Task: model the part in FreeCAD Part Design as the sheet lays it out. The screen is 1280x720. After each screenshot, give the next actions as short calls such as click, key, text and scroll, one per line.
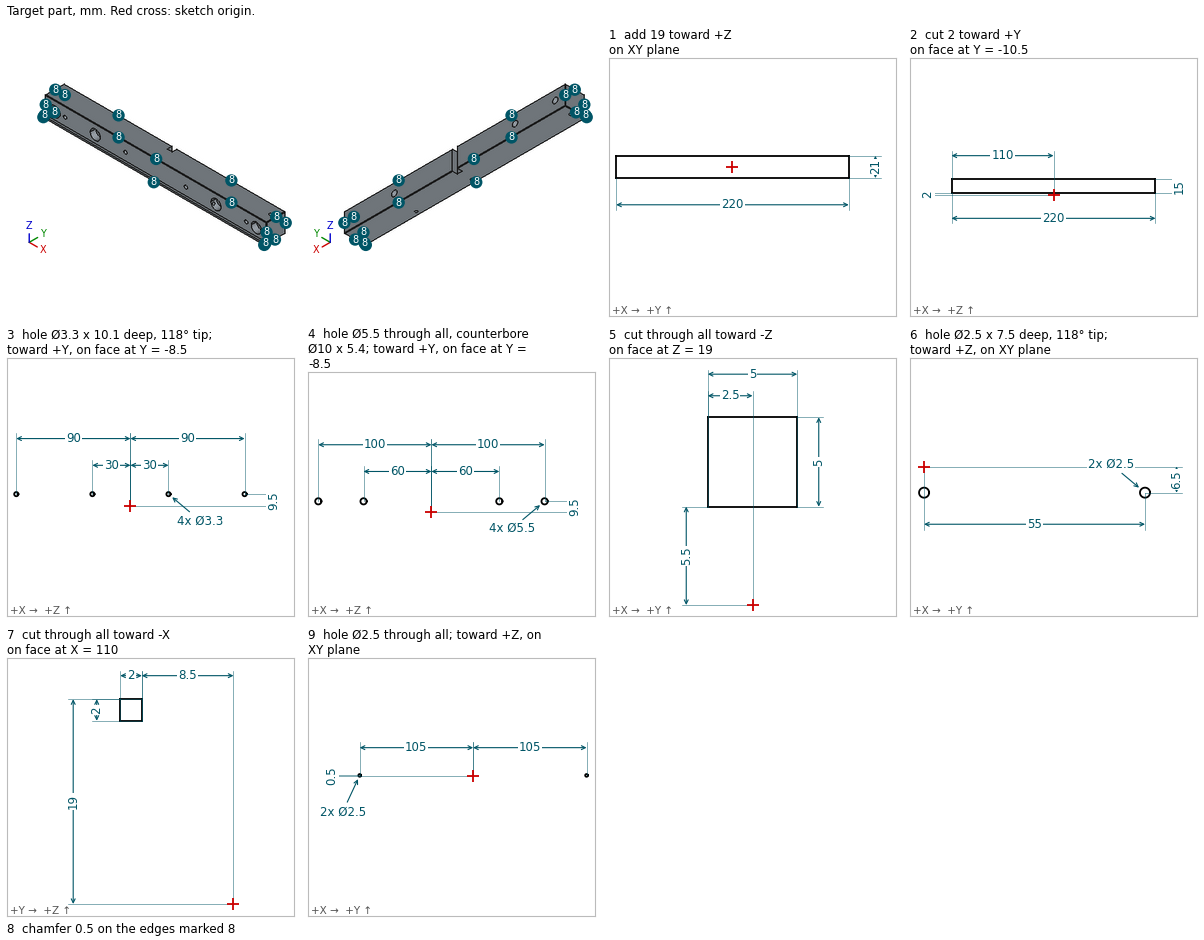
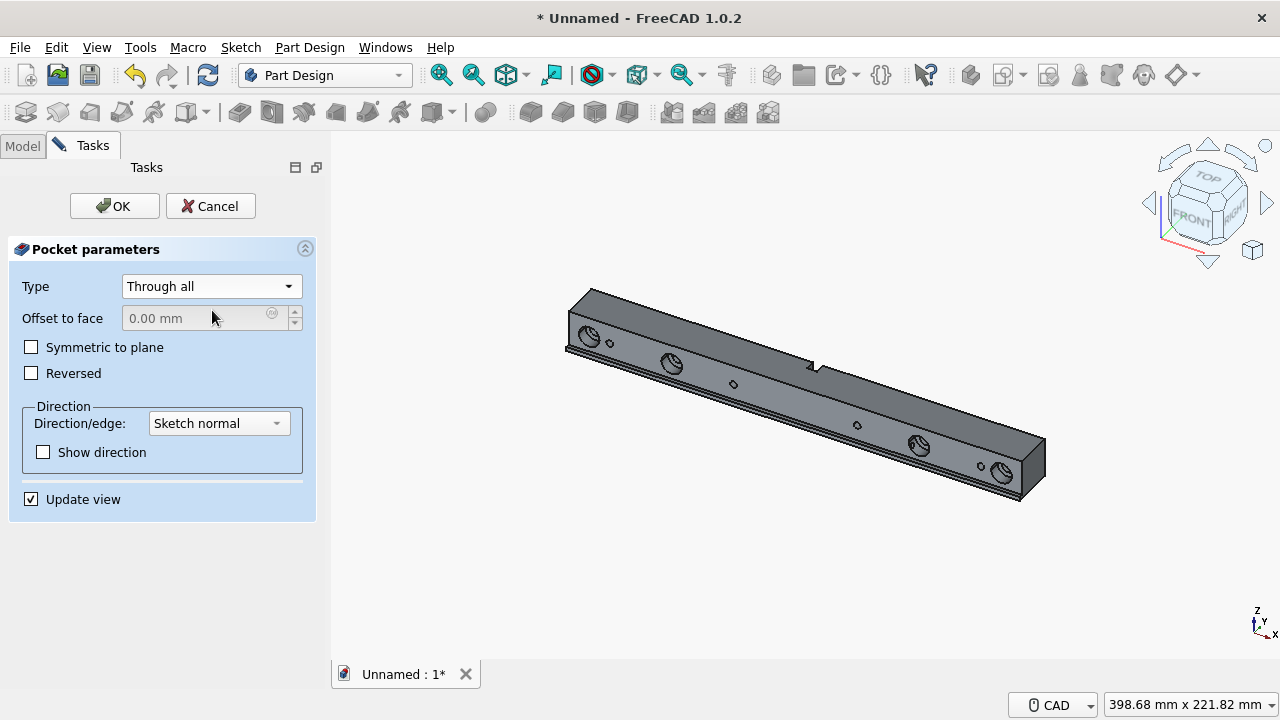
click(115, 206)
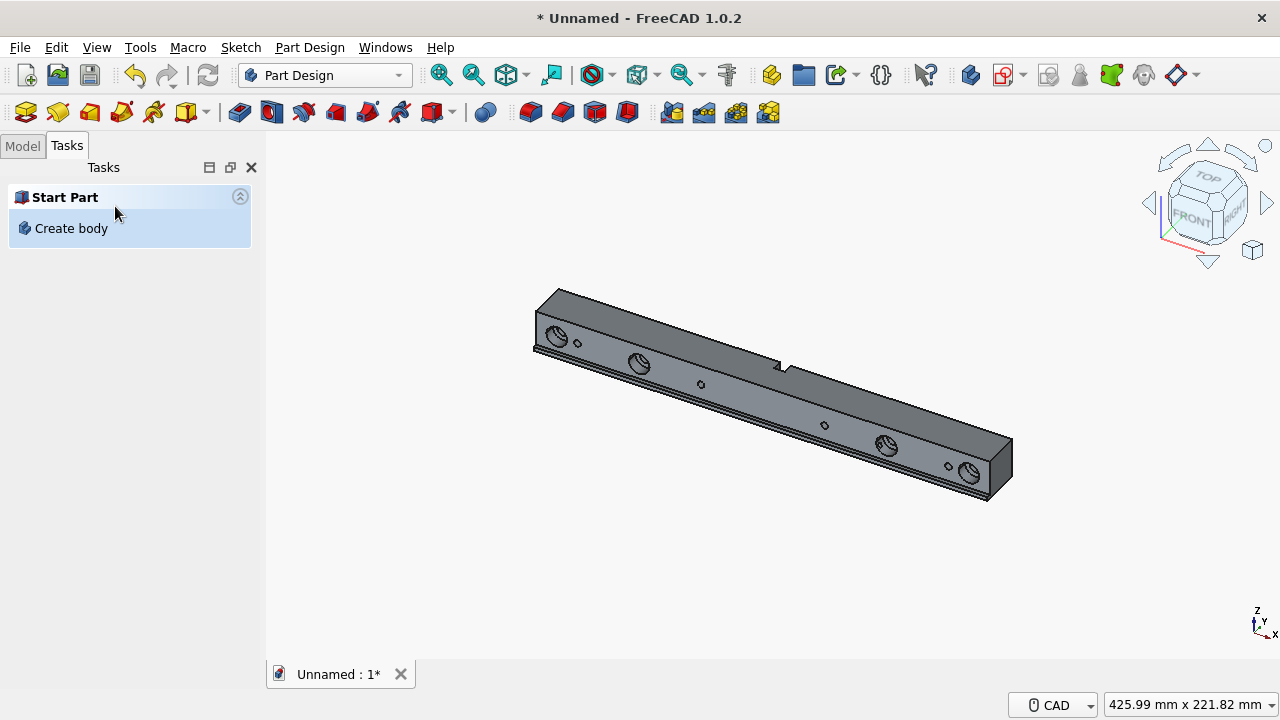
click(1000, 469)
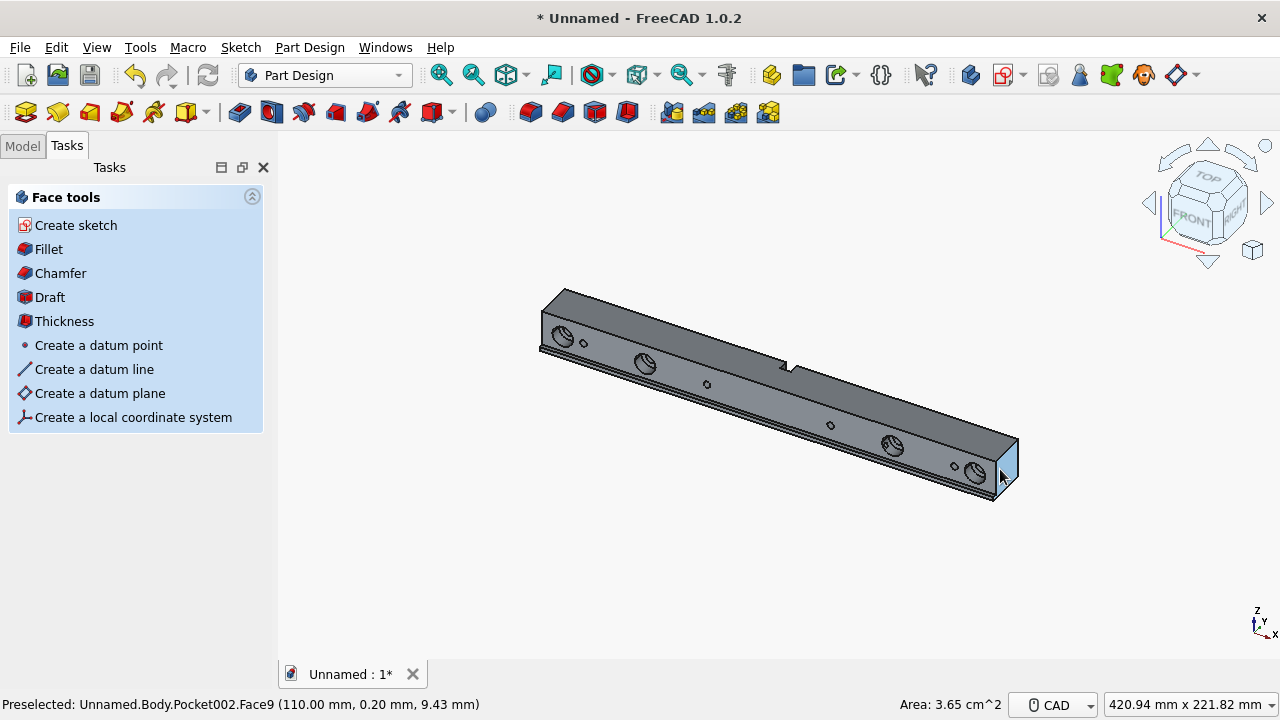
click(769, 386, ctrl)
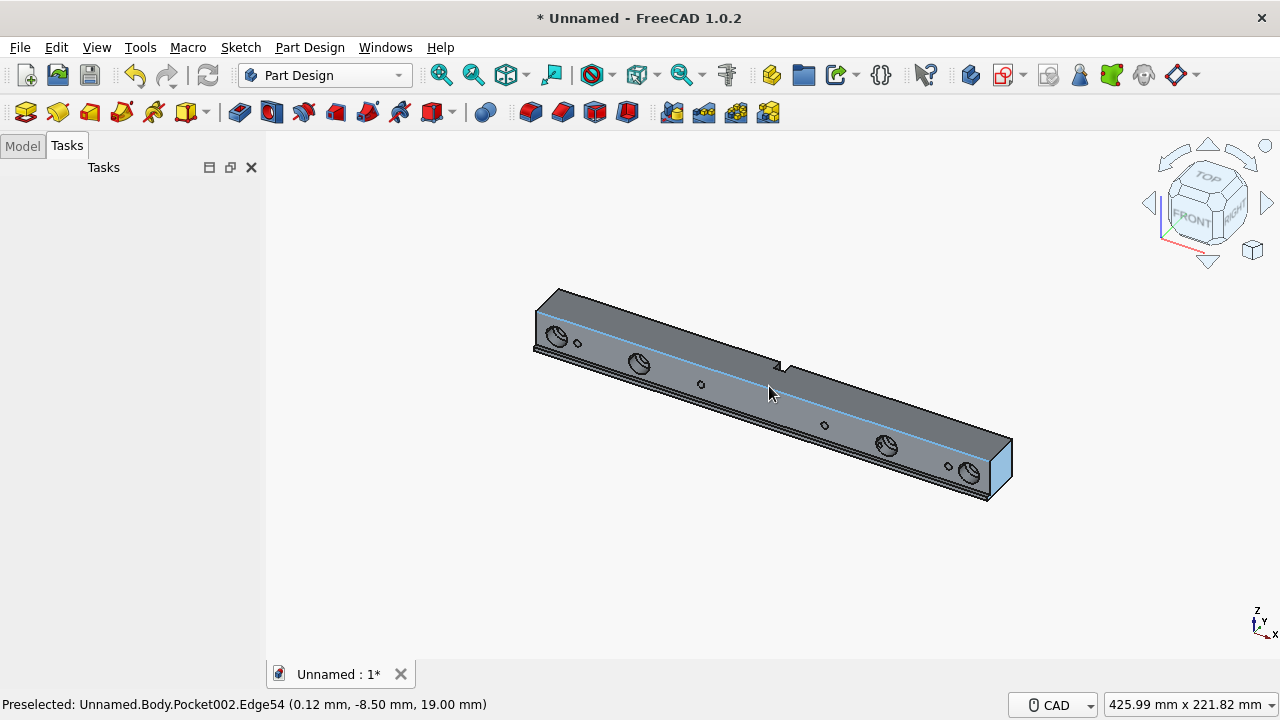
key(0)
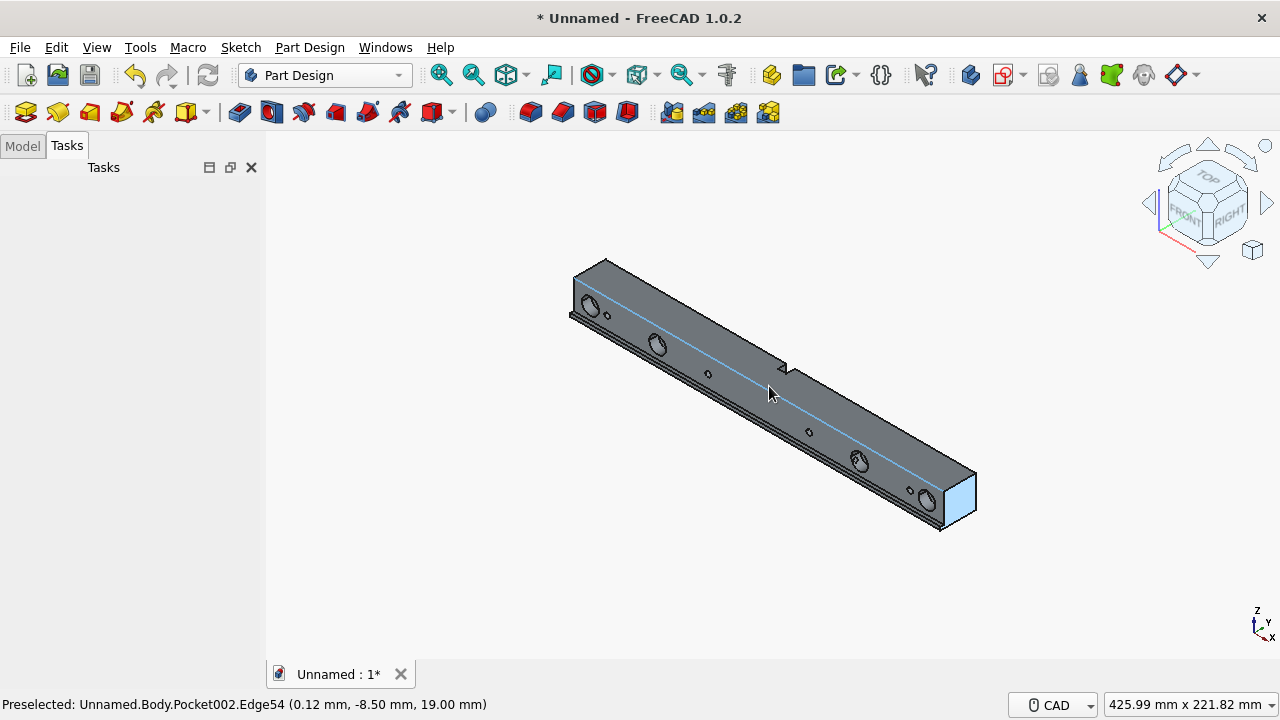
key(2)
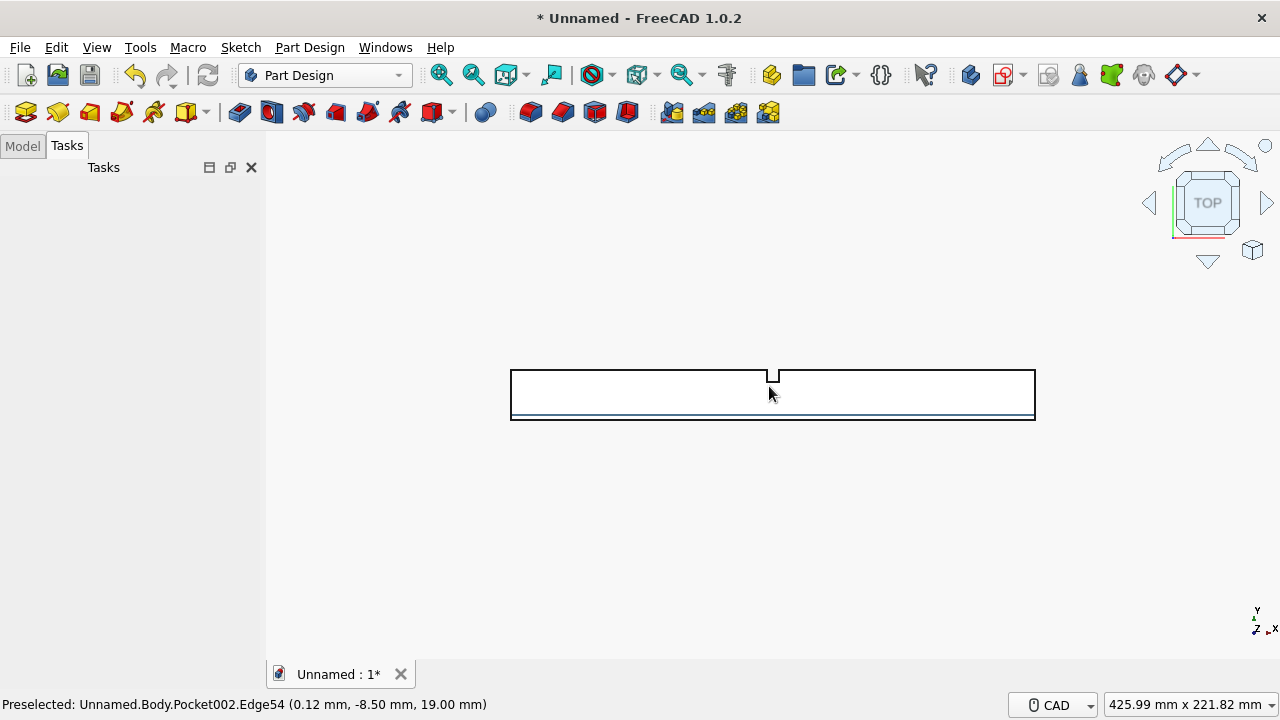
click(907, 369, ctrl)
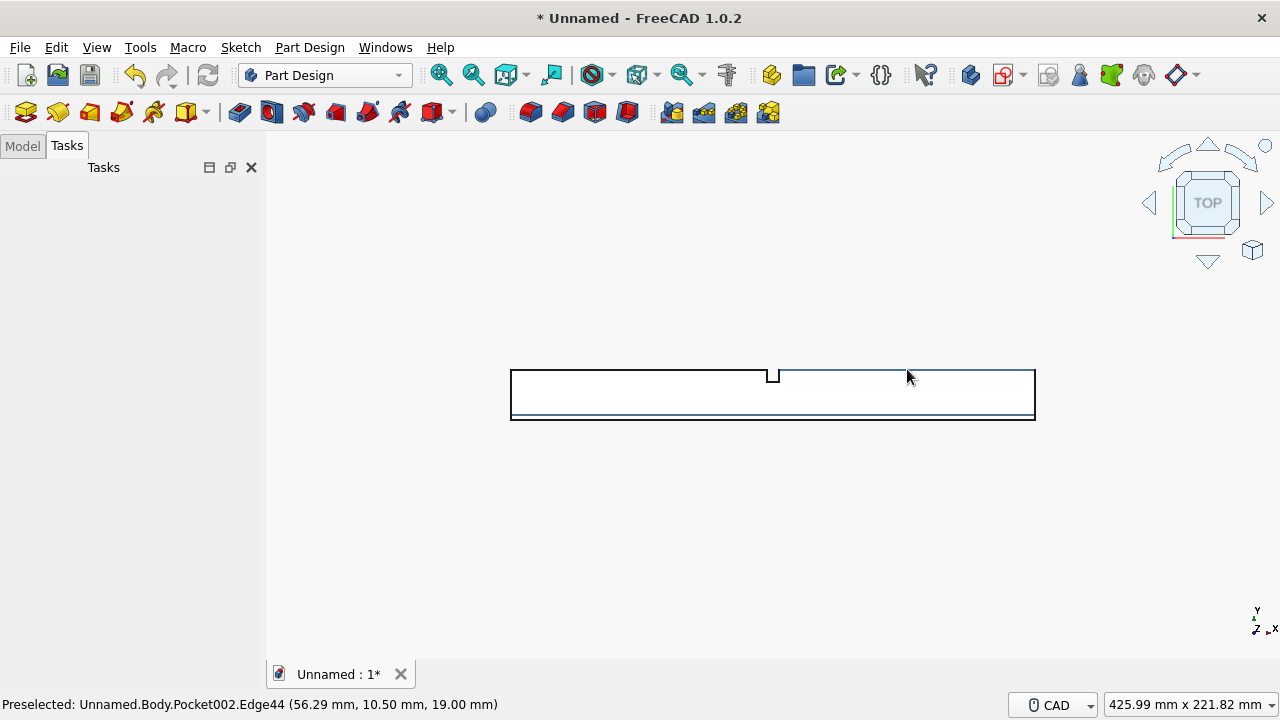
click(639, 369, ctrl)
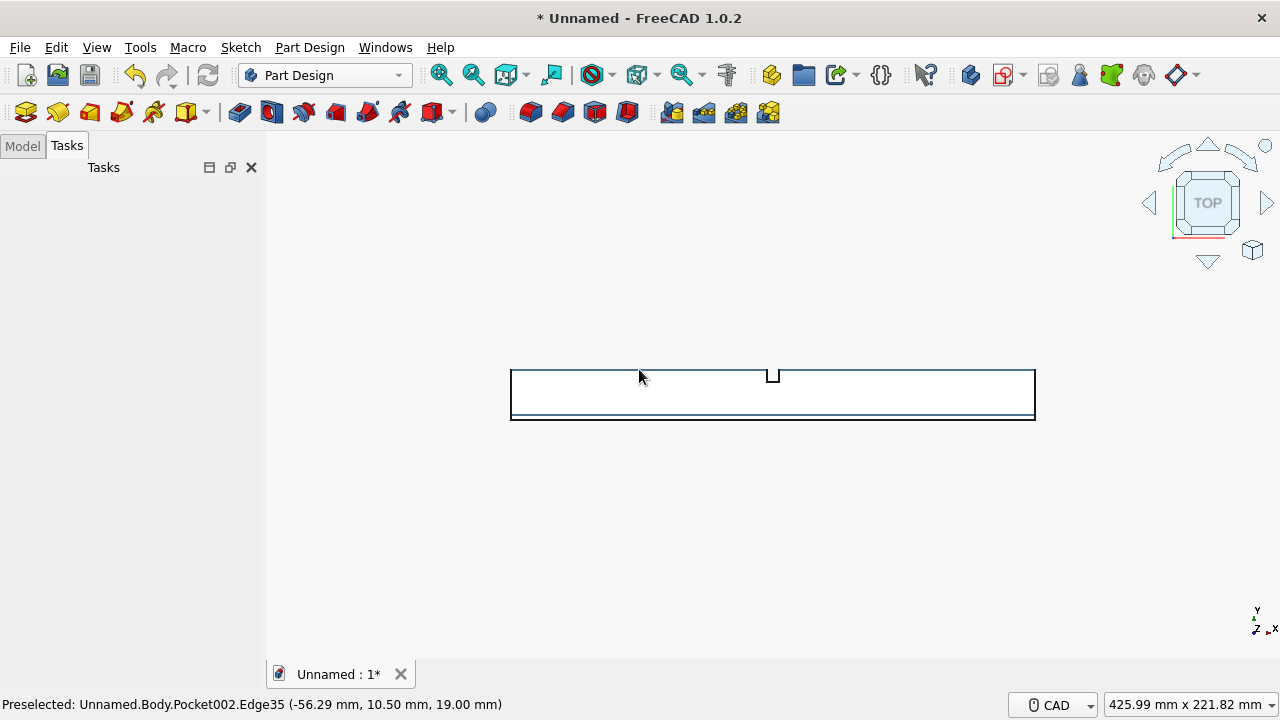
key(1)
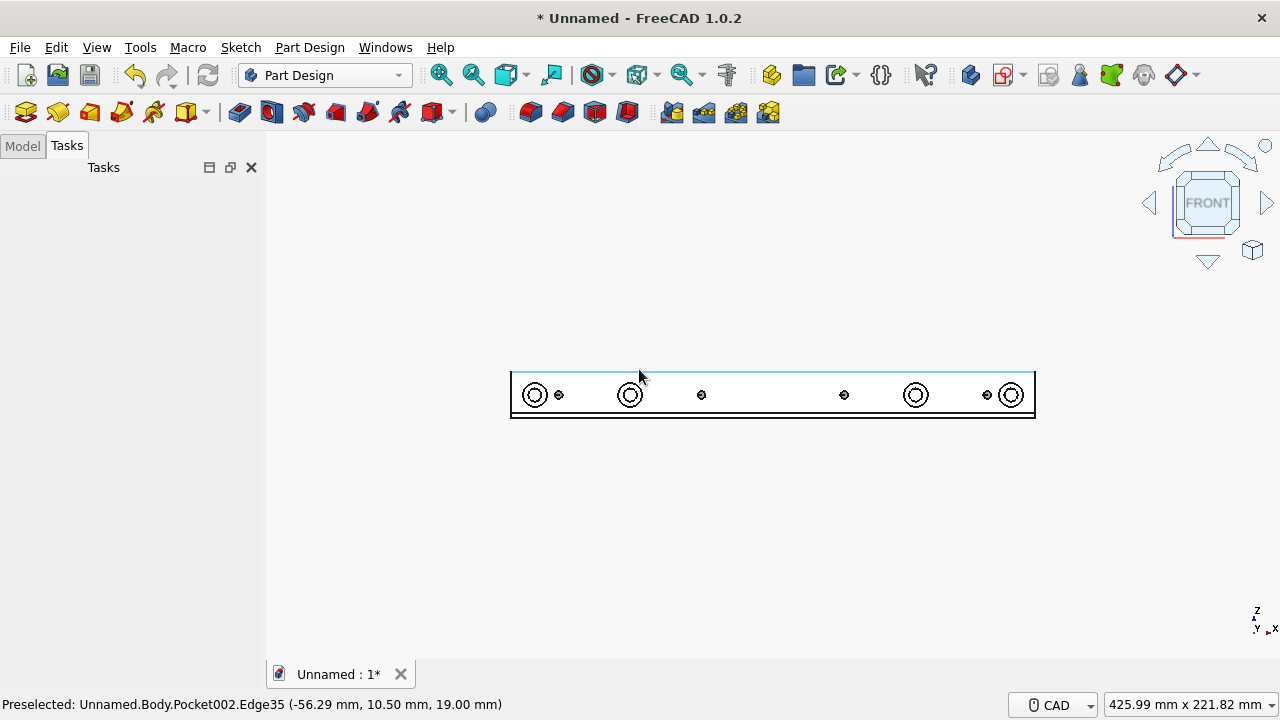
click(773, 417, ctrl)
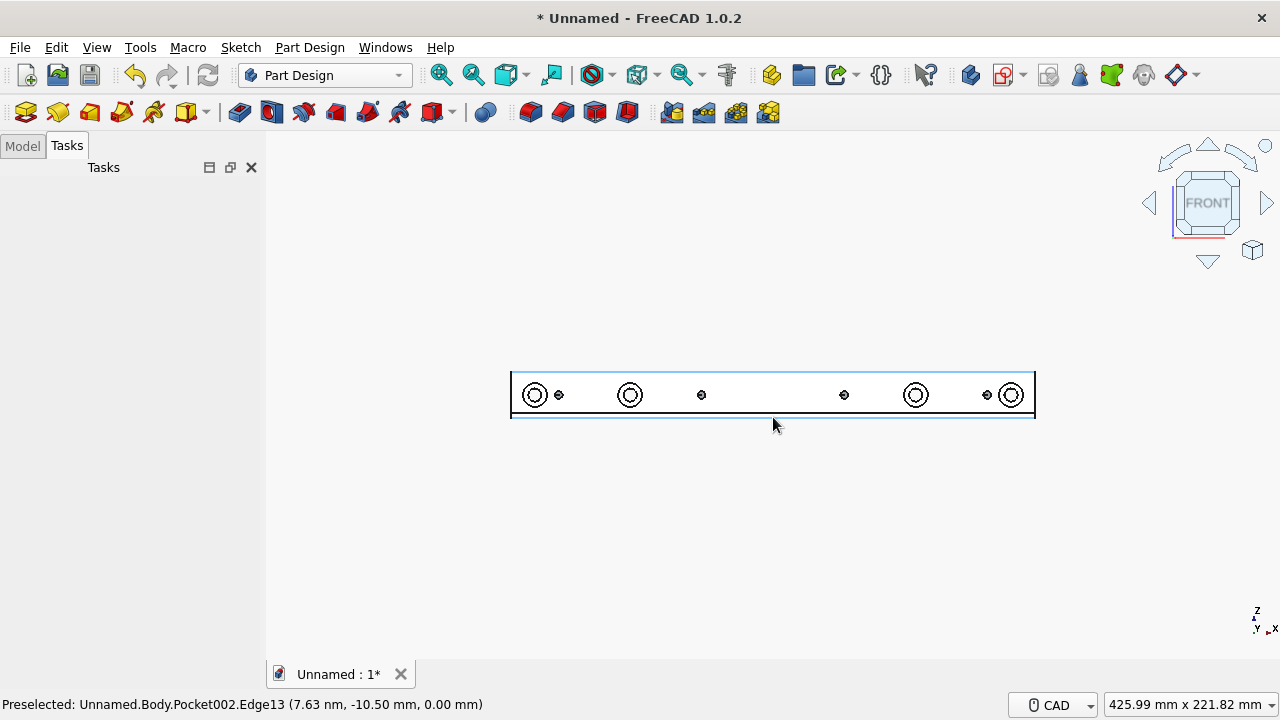
key(3)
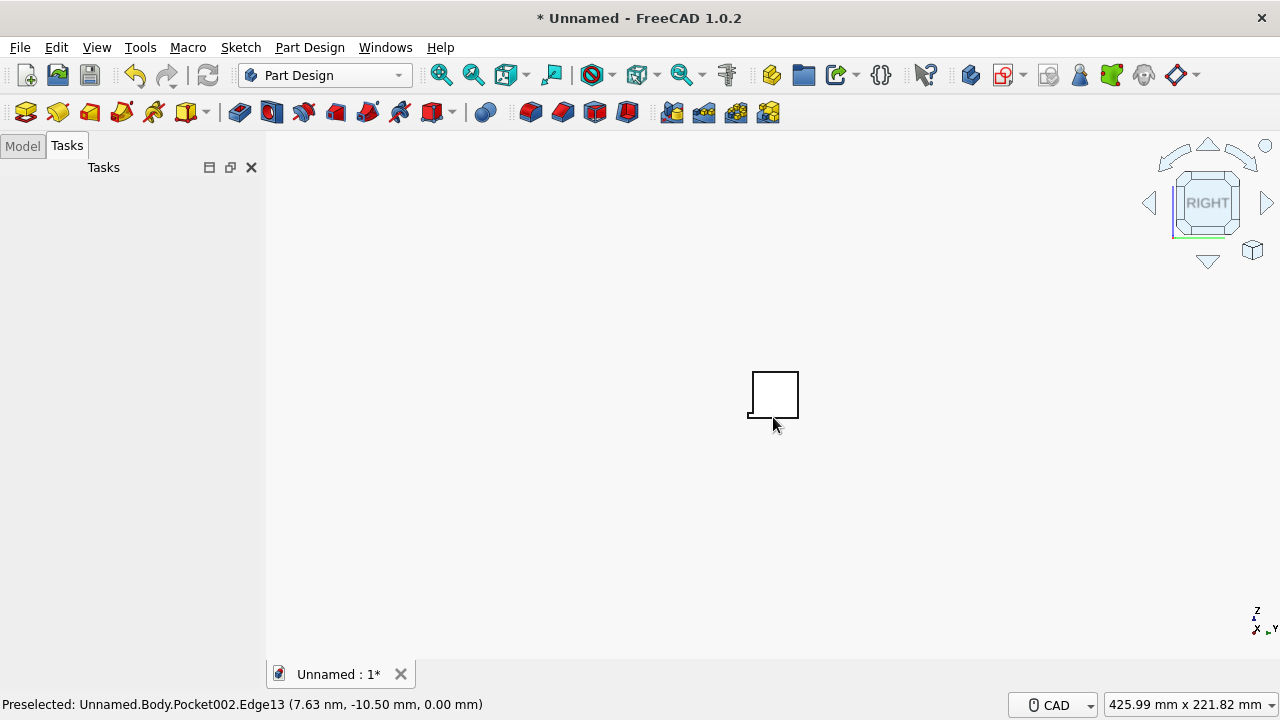
click(442, 76)